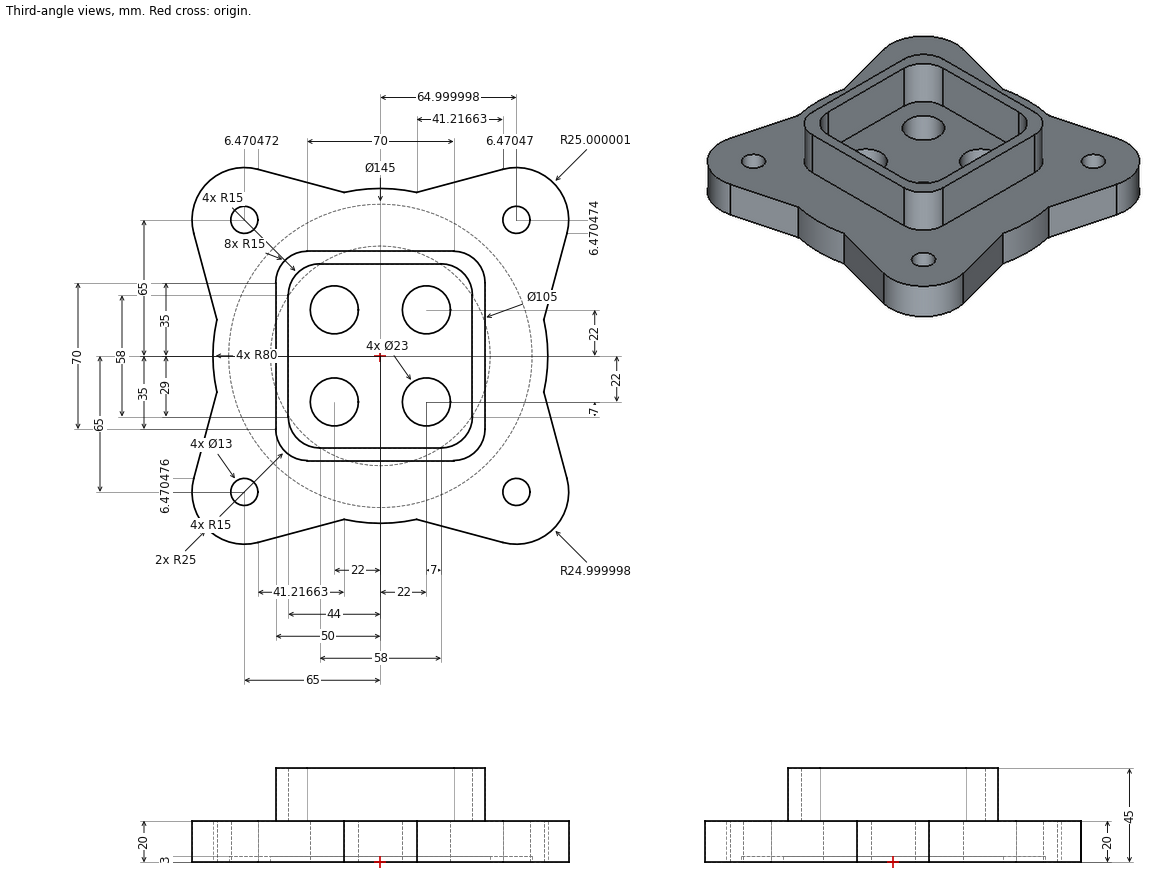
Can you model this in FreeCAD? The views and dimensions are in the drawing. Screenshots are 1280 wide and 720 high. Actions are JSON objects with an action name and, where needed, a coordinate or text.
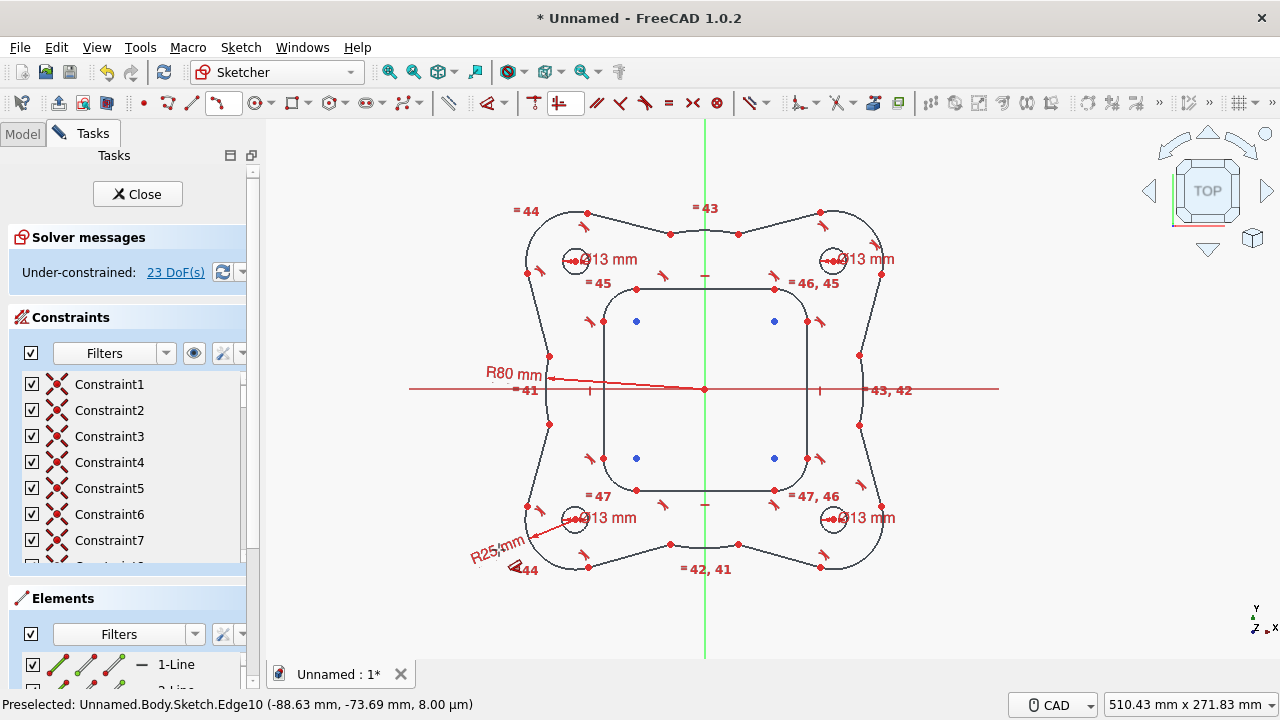
{"action": "left_click", "coordinate": [851, 566]}
{"action": "left_click", "coordinate": [862, 596]}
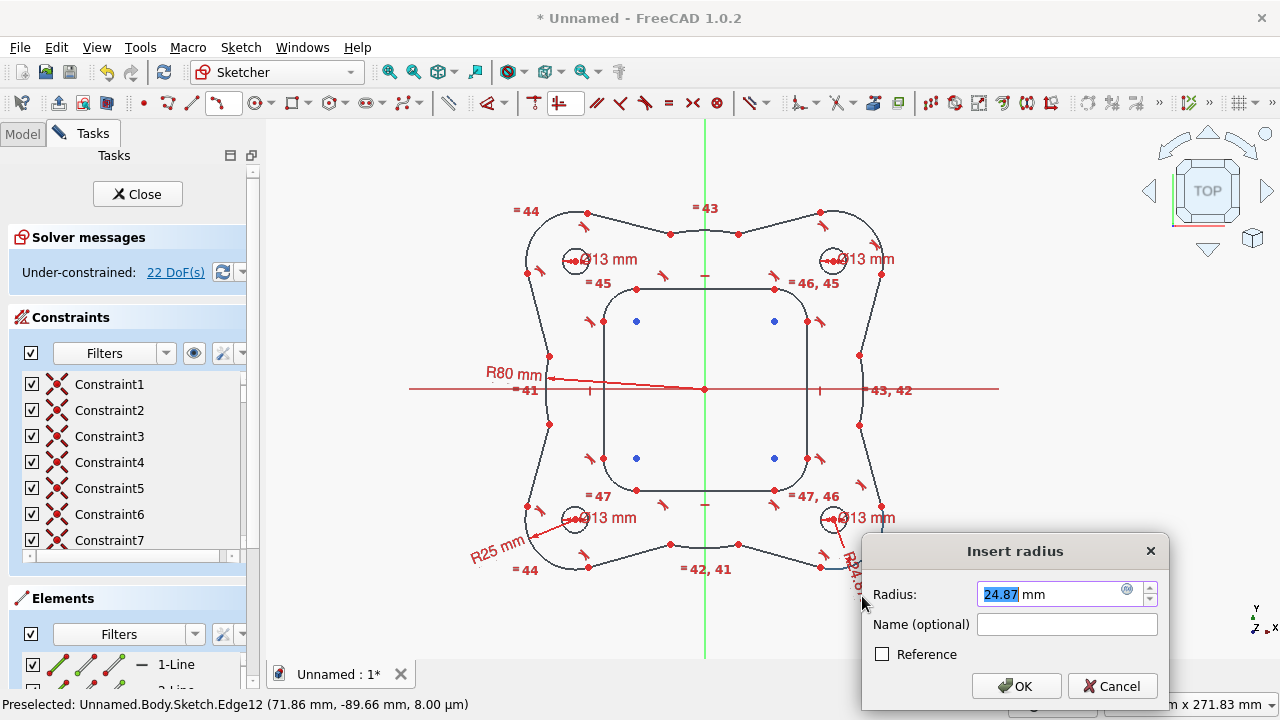
{"action": "type", "text": "24.999998"}
{"action": "key", "text": "Return"}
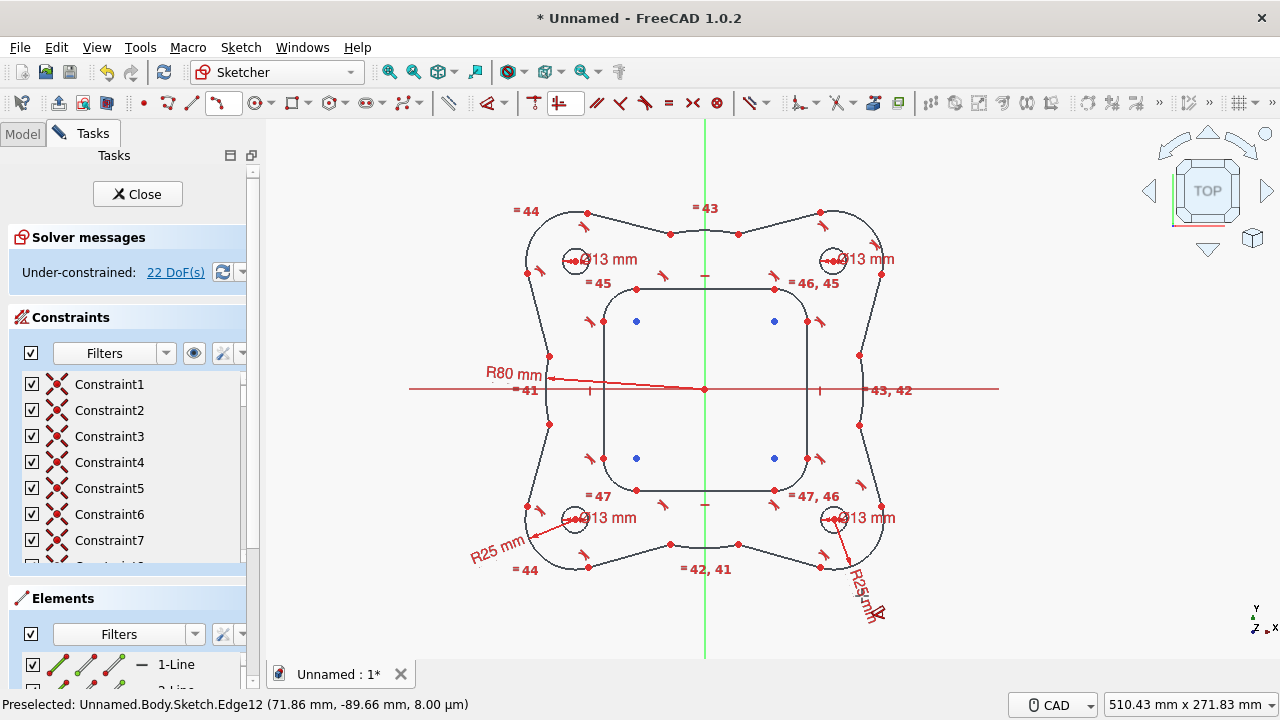
{"action": "left_click", "coordinate": [880, 243]}
{"action": "left_click", "coordinate": [910, 231]}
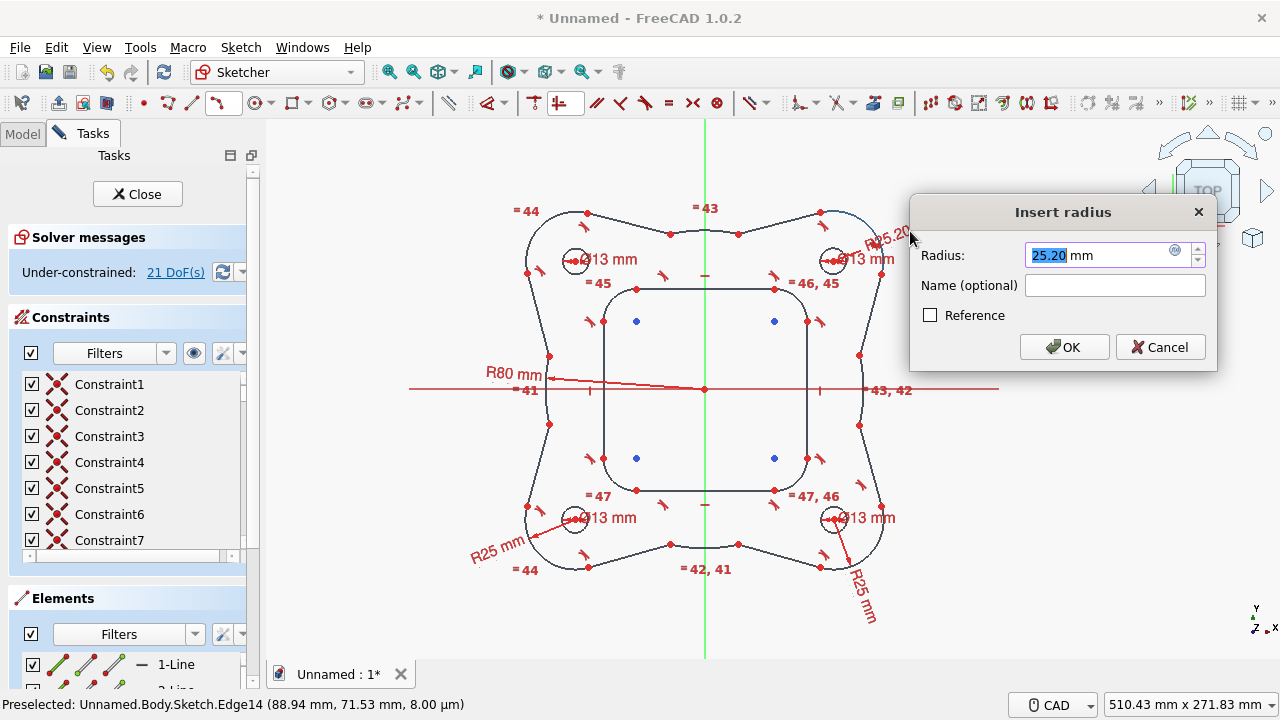
{"action": "type", "text": "25.000001"}
{"action": "key", "text": "Return"}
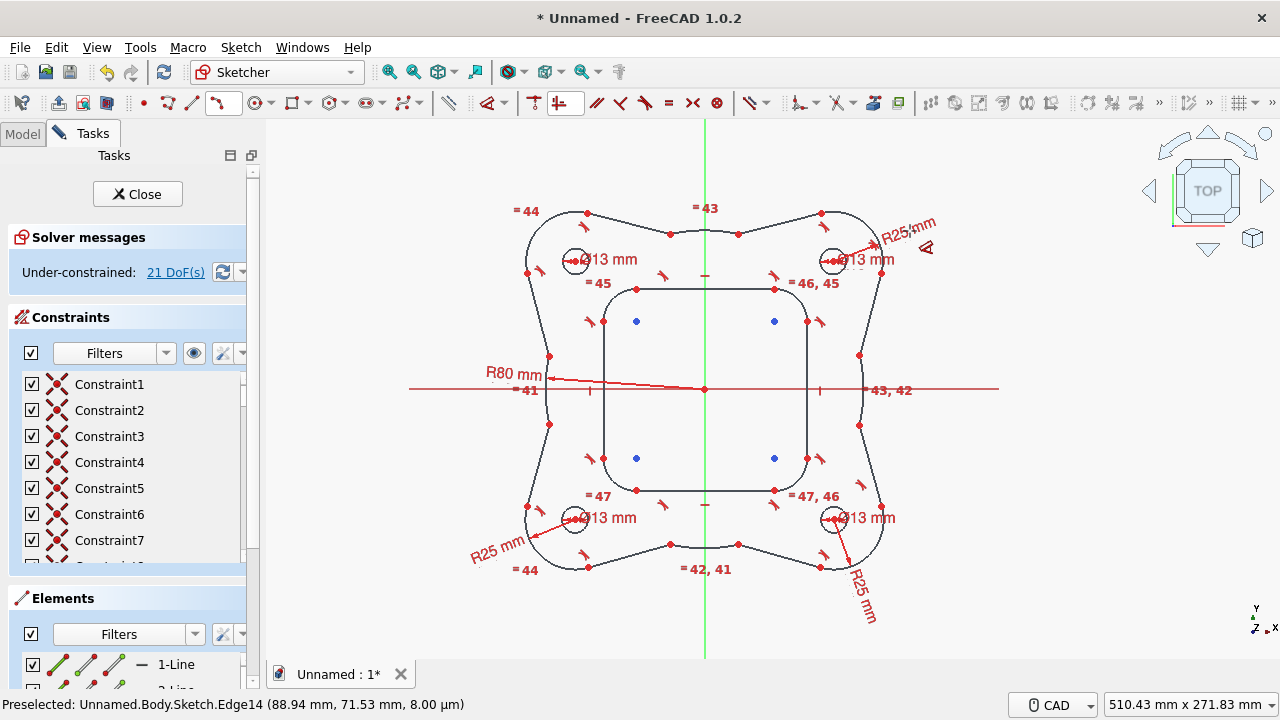
{"action": "scroll", "coordinate": [621, 293], "scroll_direction": "up", "scroll_amount": 2}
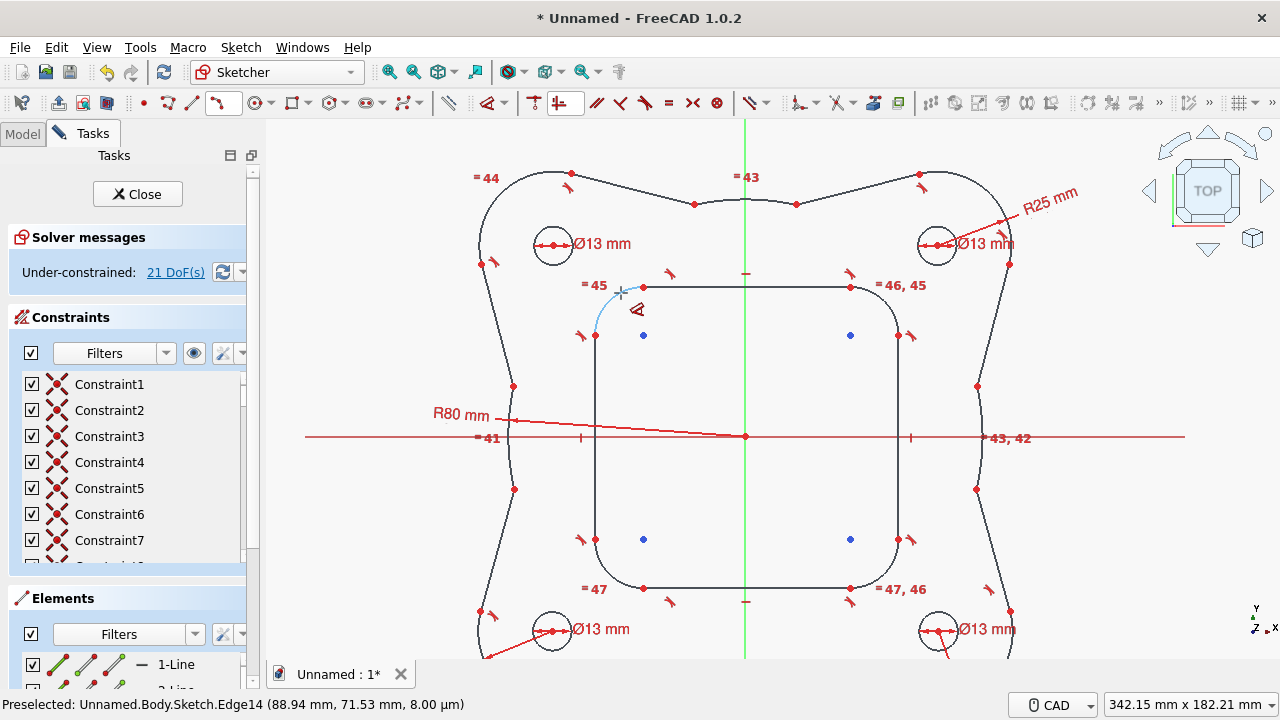
{"action": "left_click", "coordinate": [621, 292]}
{"action": "left_click", "coordinate": [606, 264]}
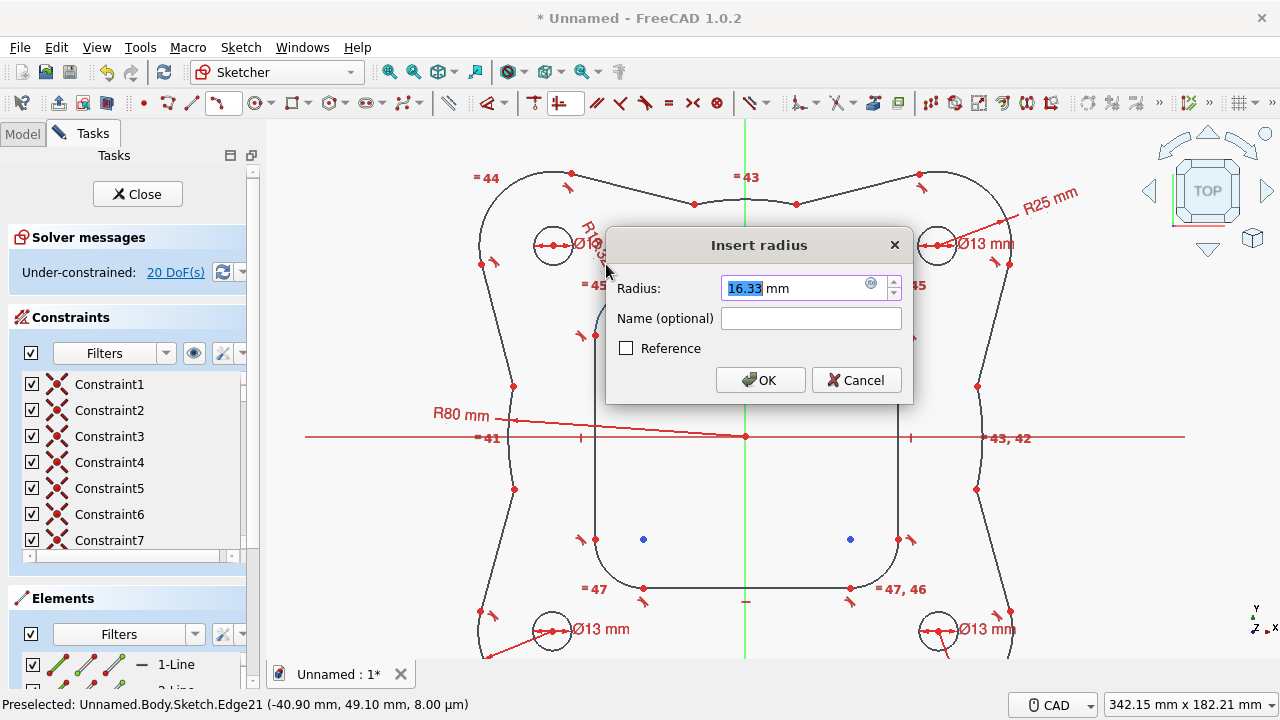
{"action": "type", "text": "15"}
{"action": "key", "text": "Return"}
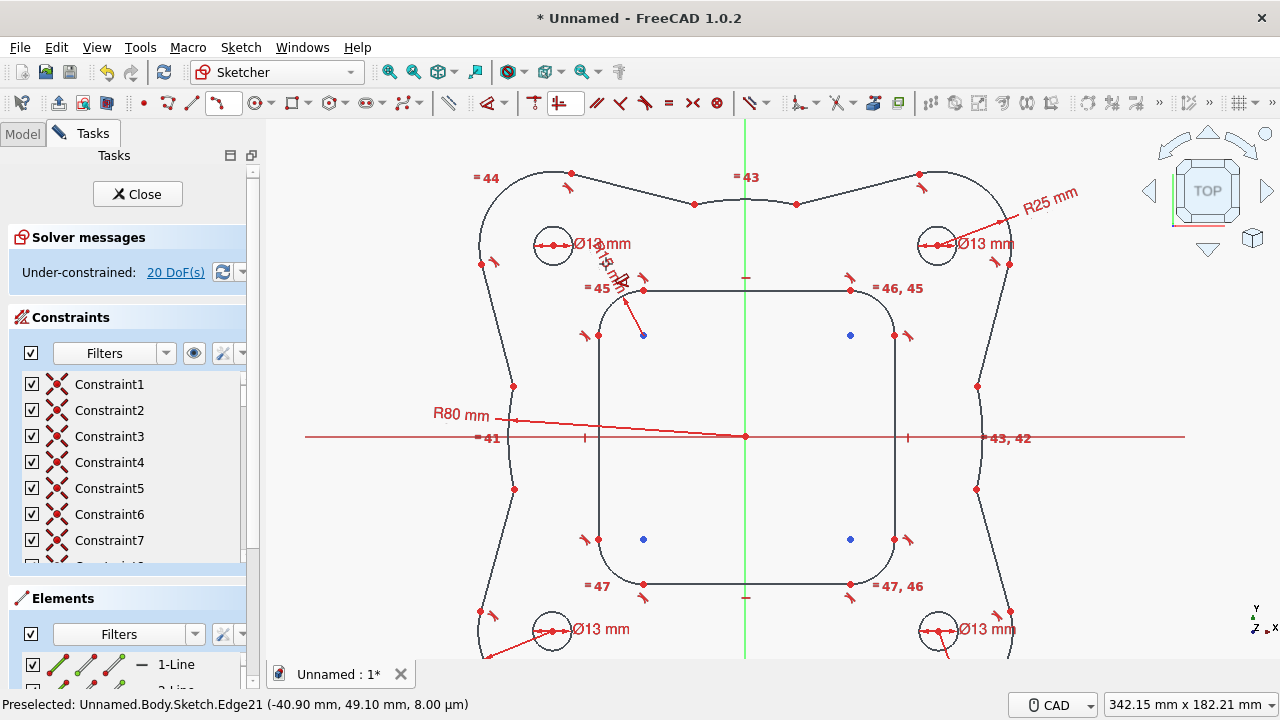
{"action": "left_click", "coordinate": [599, 478]}
{"action": "left_click", "coordinate": [565, 391]}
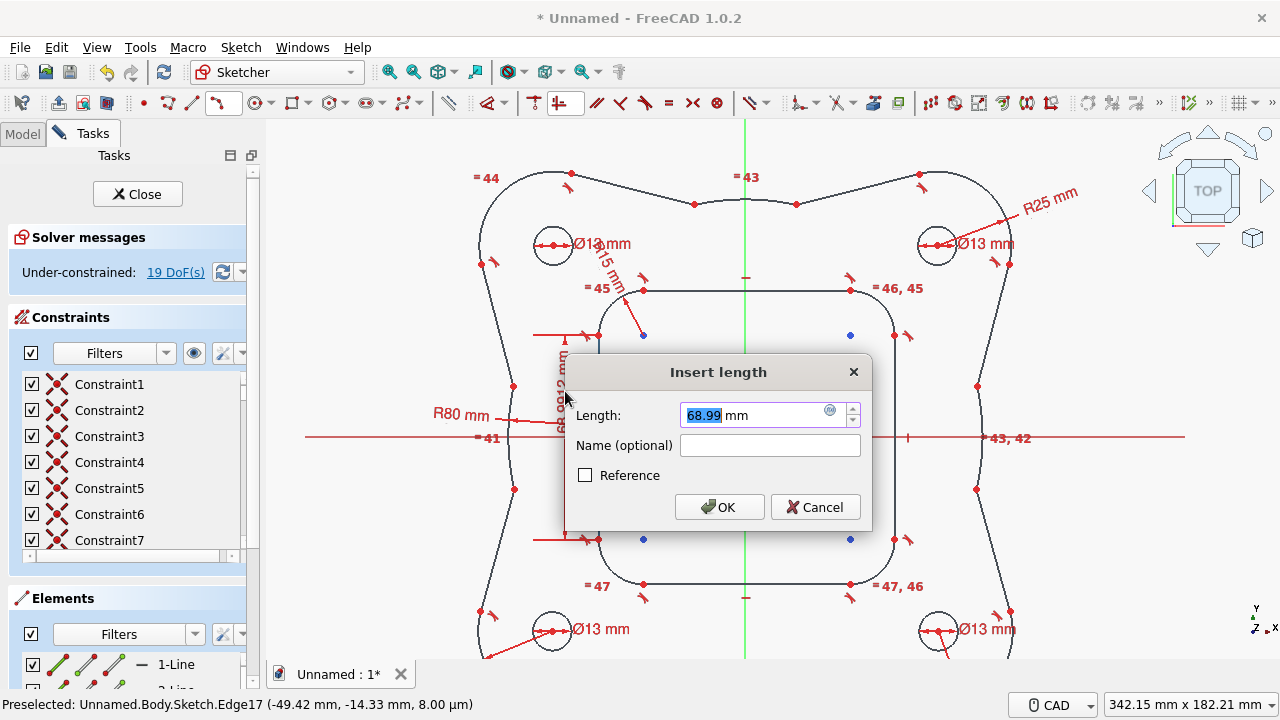
{"action": "type", "text": "70"}
{"action": "key", "text": "Return"}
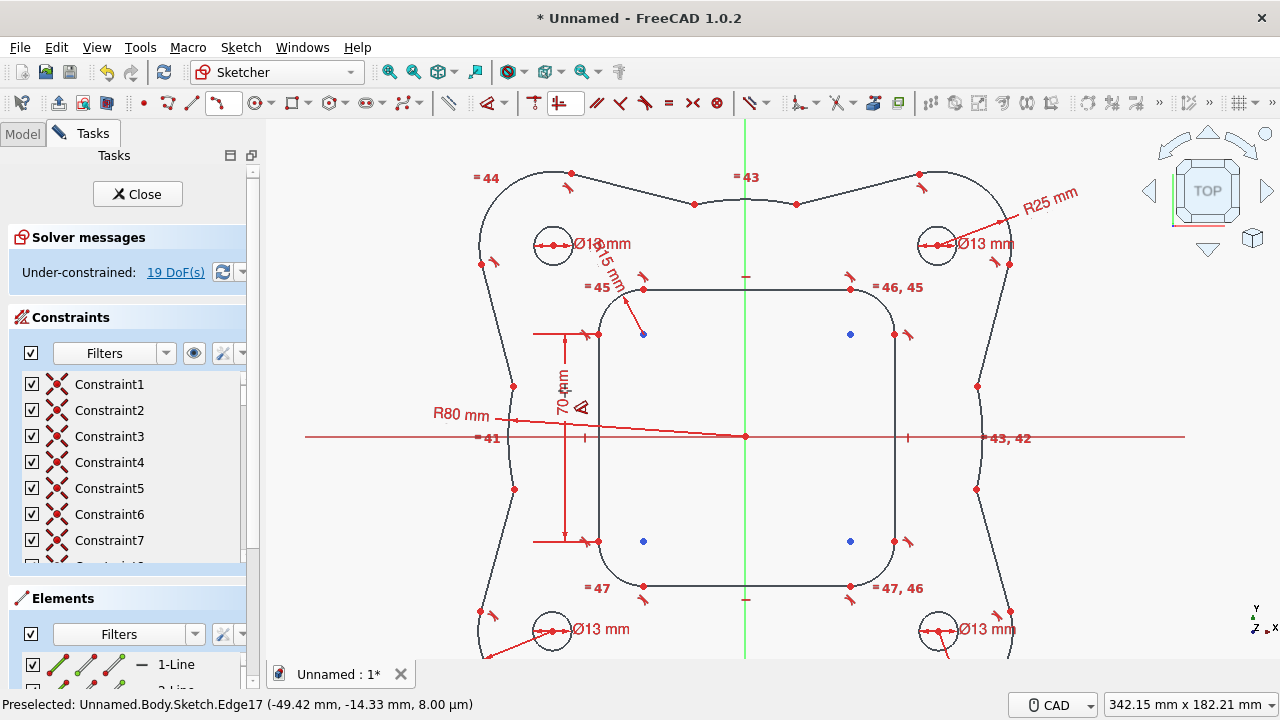
{"action": "left_click", "coordinate": [705, 290]}
{"action": "left_click", "coordinate": [699, 256]}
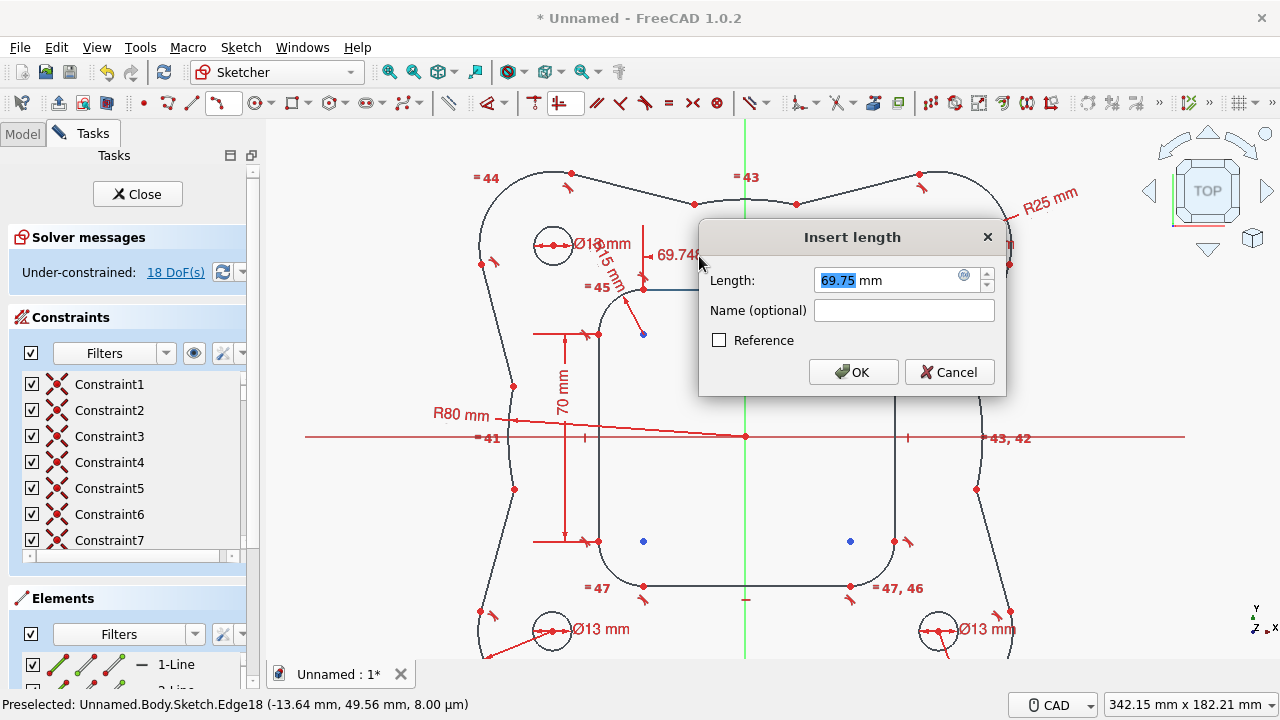
{"action": "type", "text": "70"}
{"action": "key", "text": "Return"}